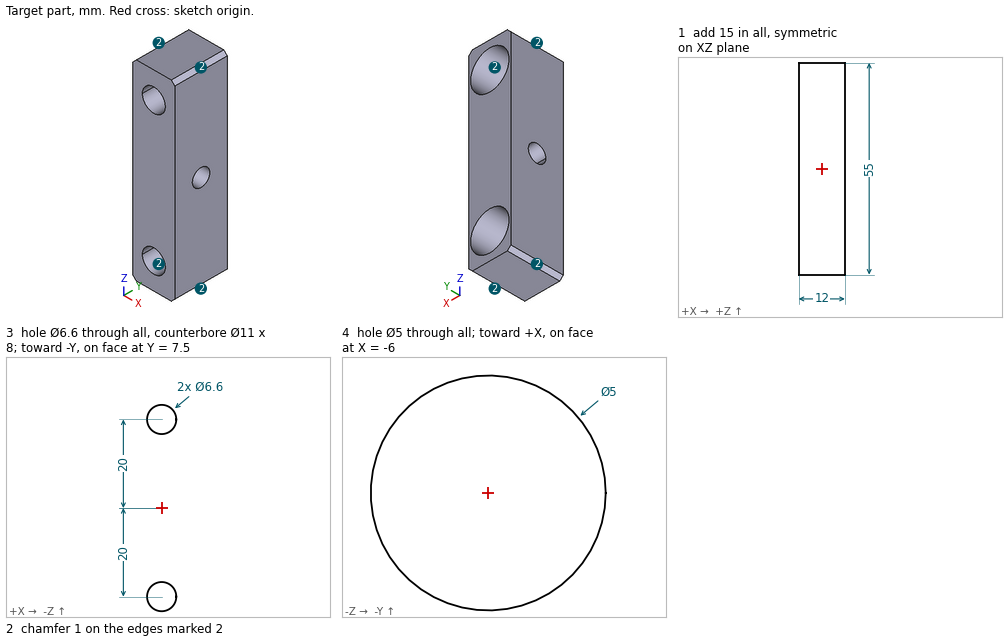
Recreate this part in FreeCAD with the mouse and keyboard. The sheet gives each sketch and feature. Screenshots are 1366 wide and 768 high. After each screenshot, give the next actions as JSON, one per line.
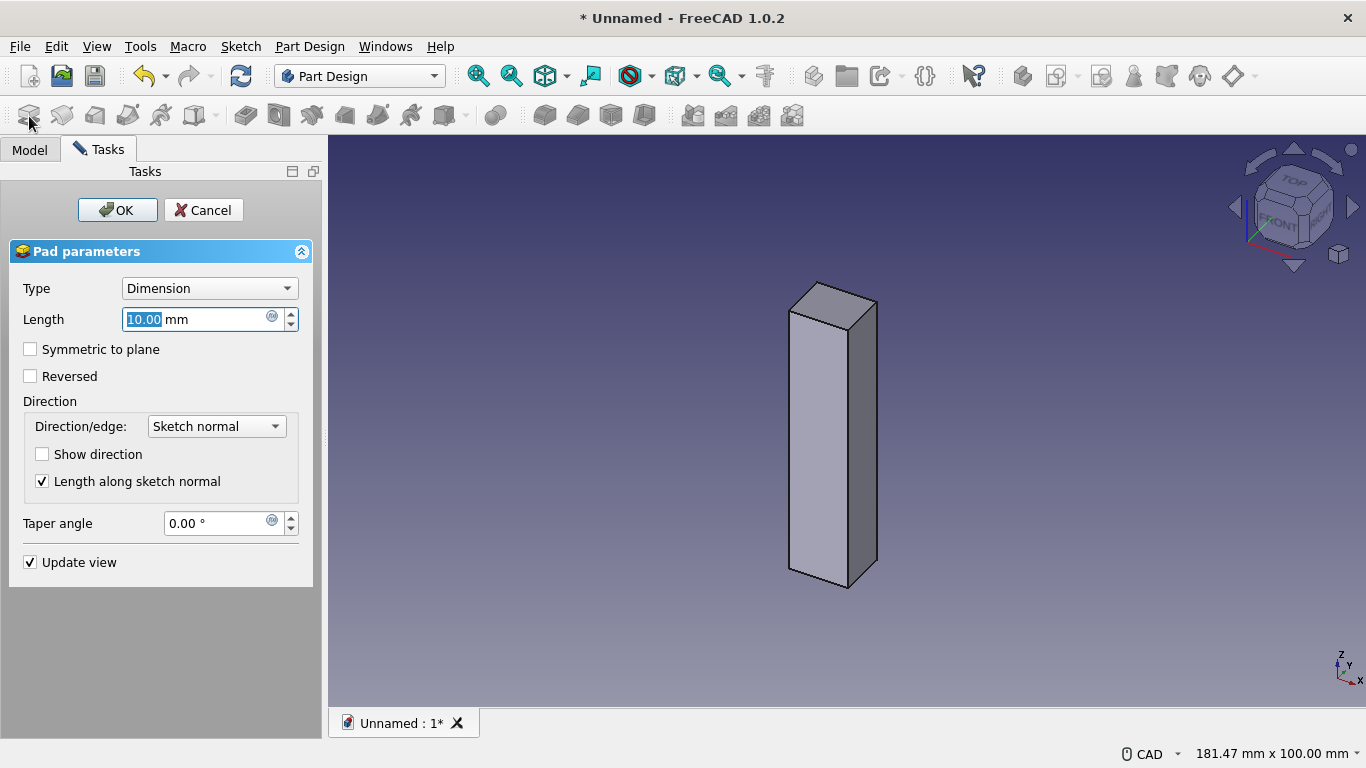
{"action": "type", "text": "15"}
{"action": "key", "text": "Tab"}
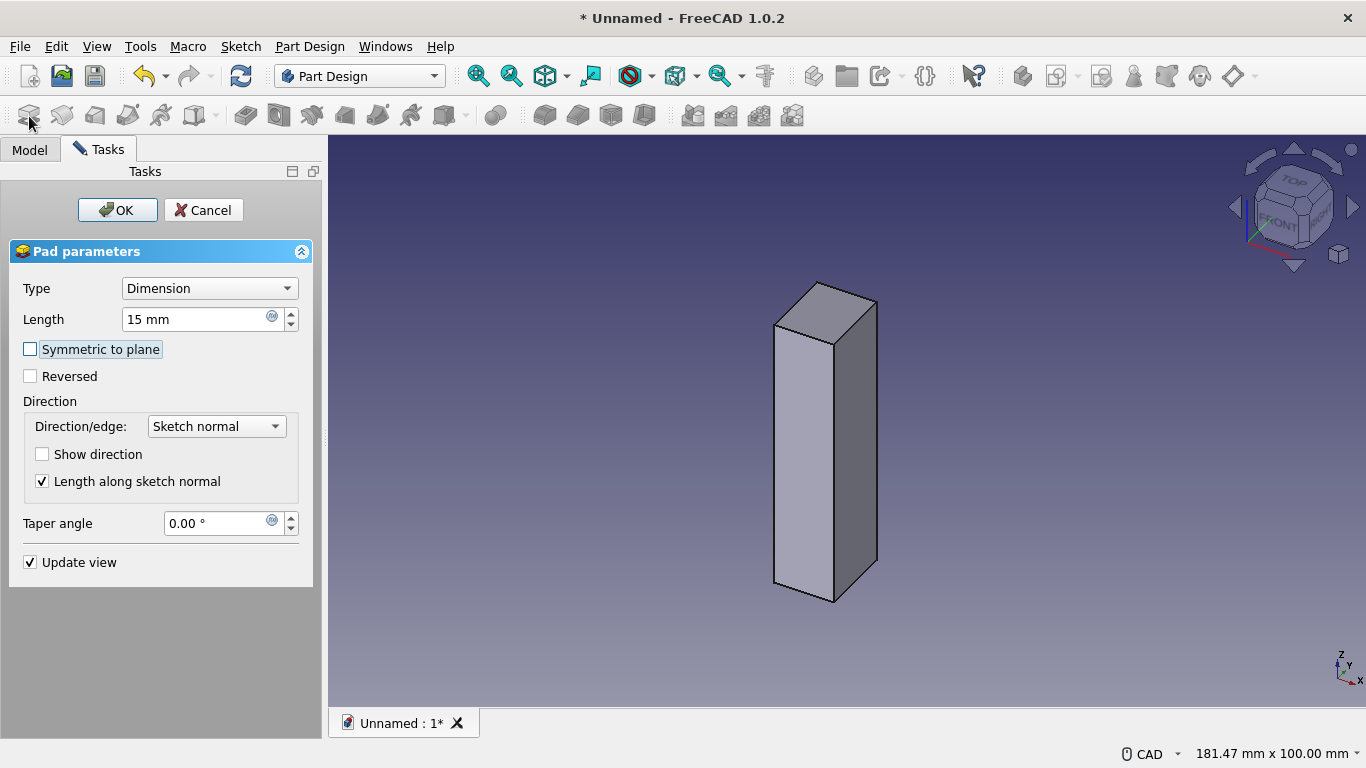
{"action": "left_click", "coordinate": [31, 349]}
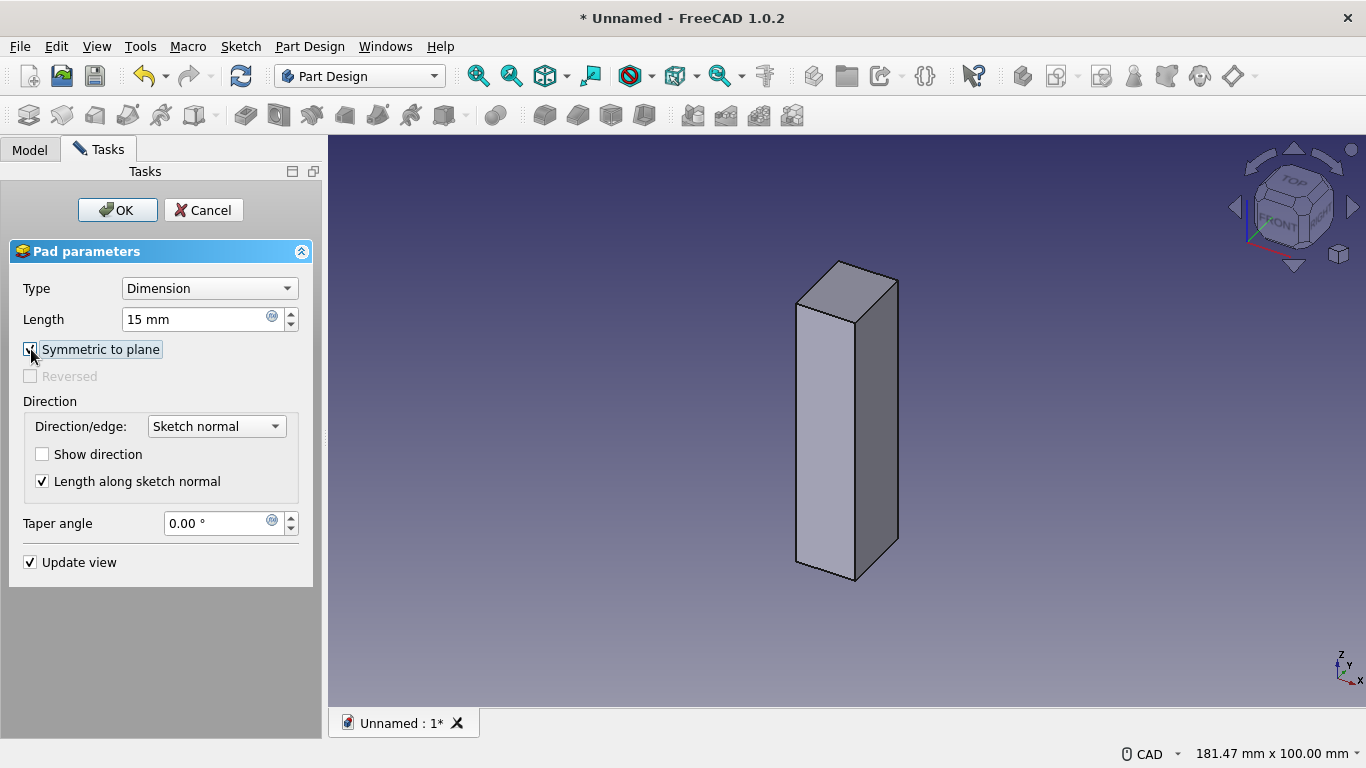
{"action": "left_click", "coordinate": [118, 210]}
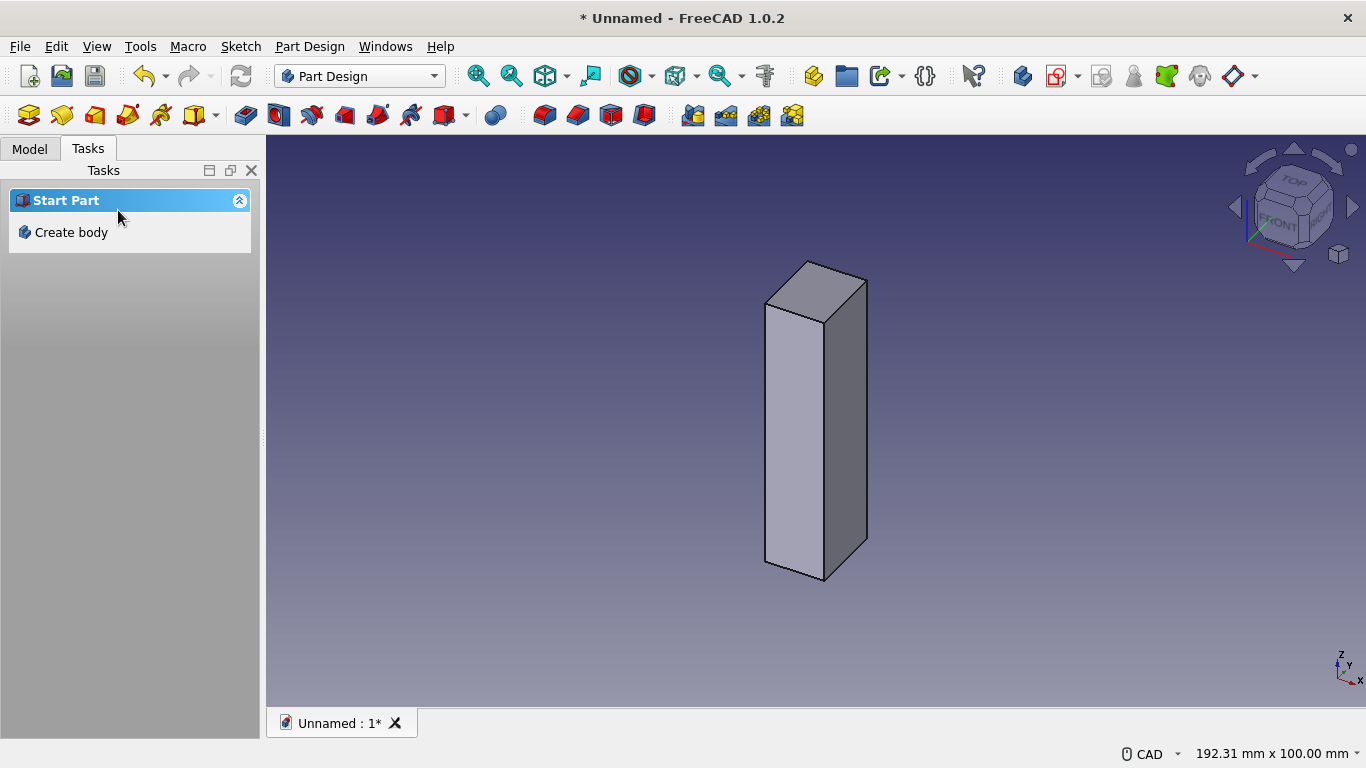
{"action": "left_click", "coordinate": [846, 301]}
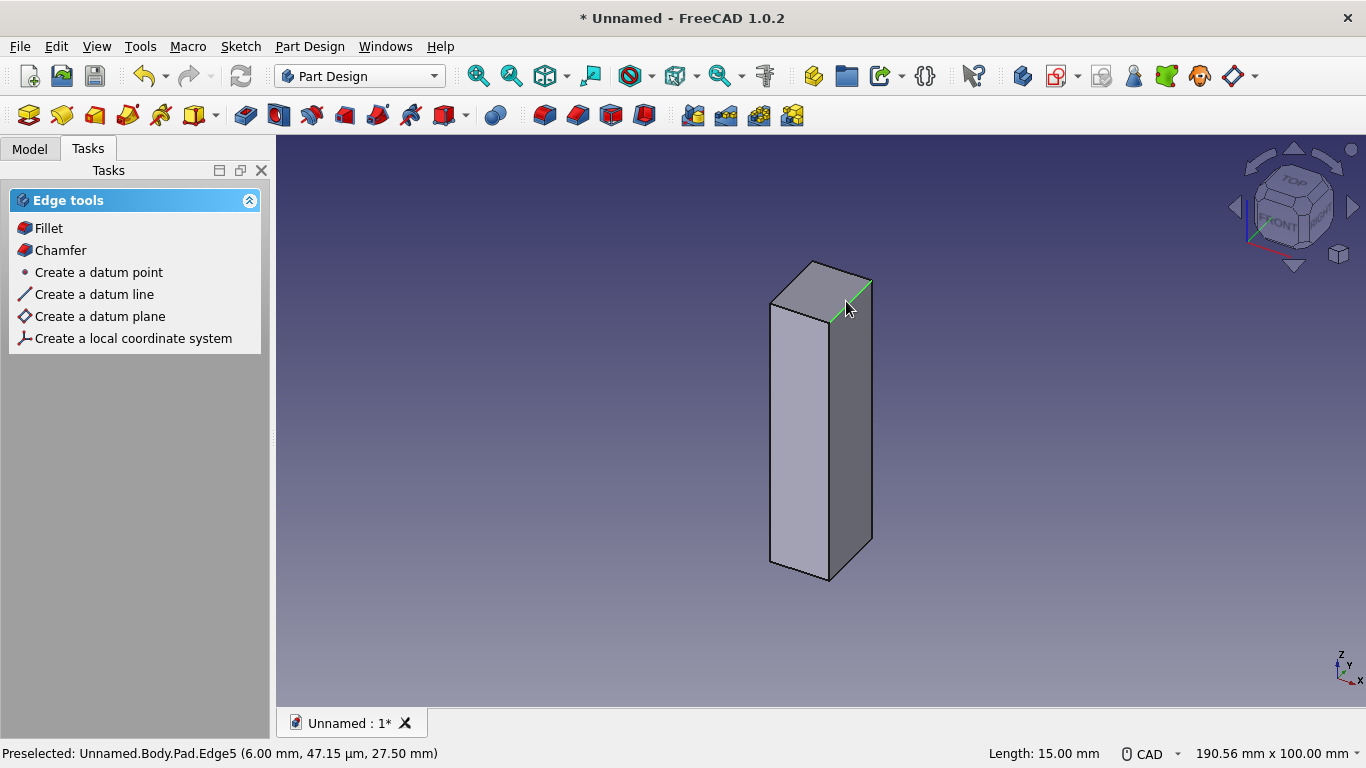
{"action": "key", "text": "0"}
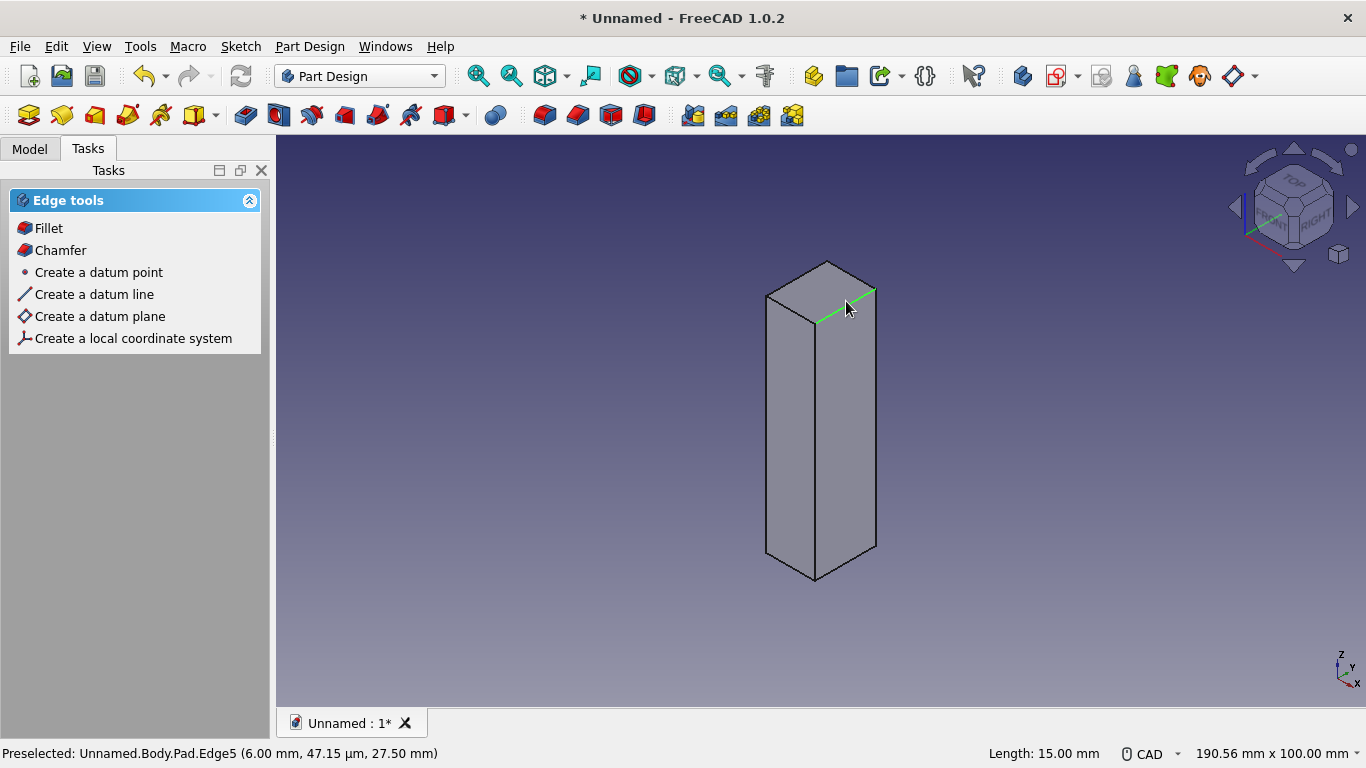
{"action": "key", "text": "2"}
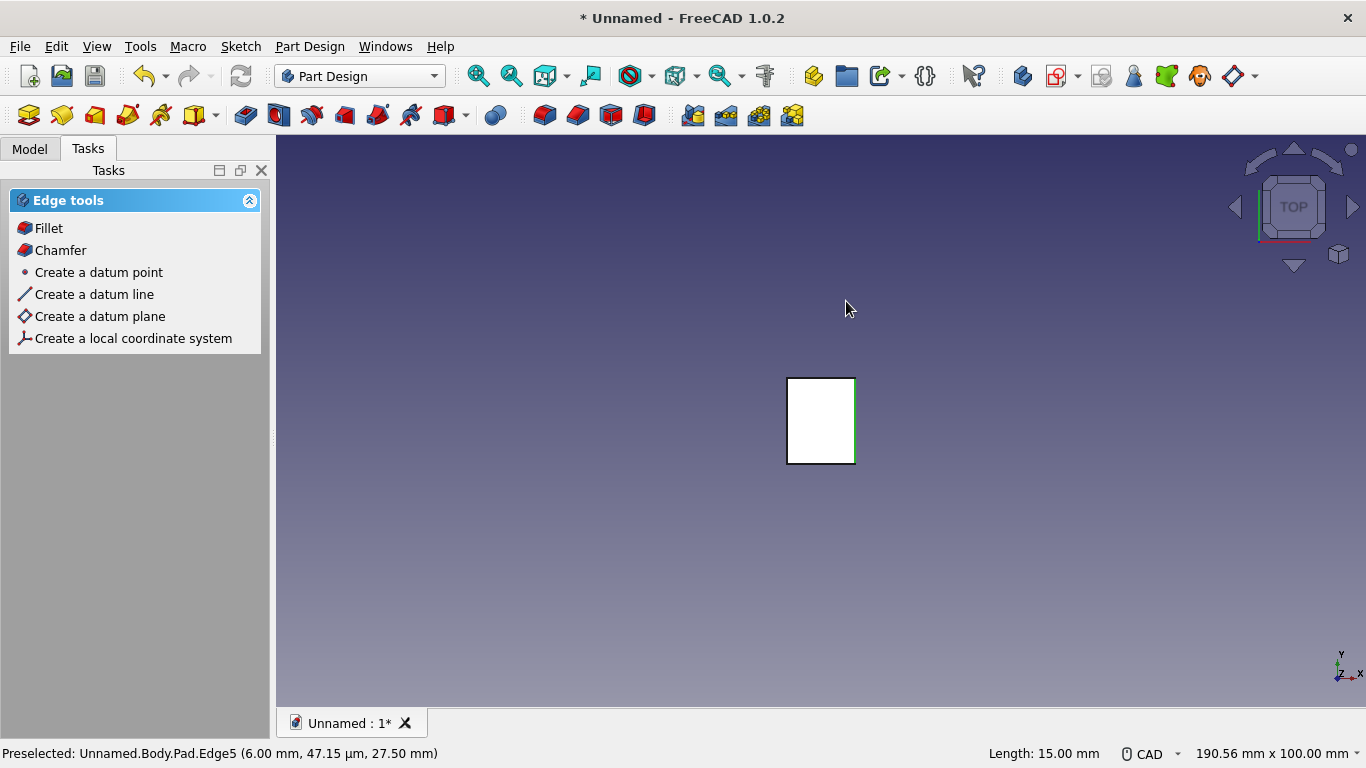
{"action": "left_click", "coordinate": [479, 76]}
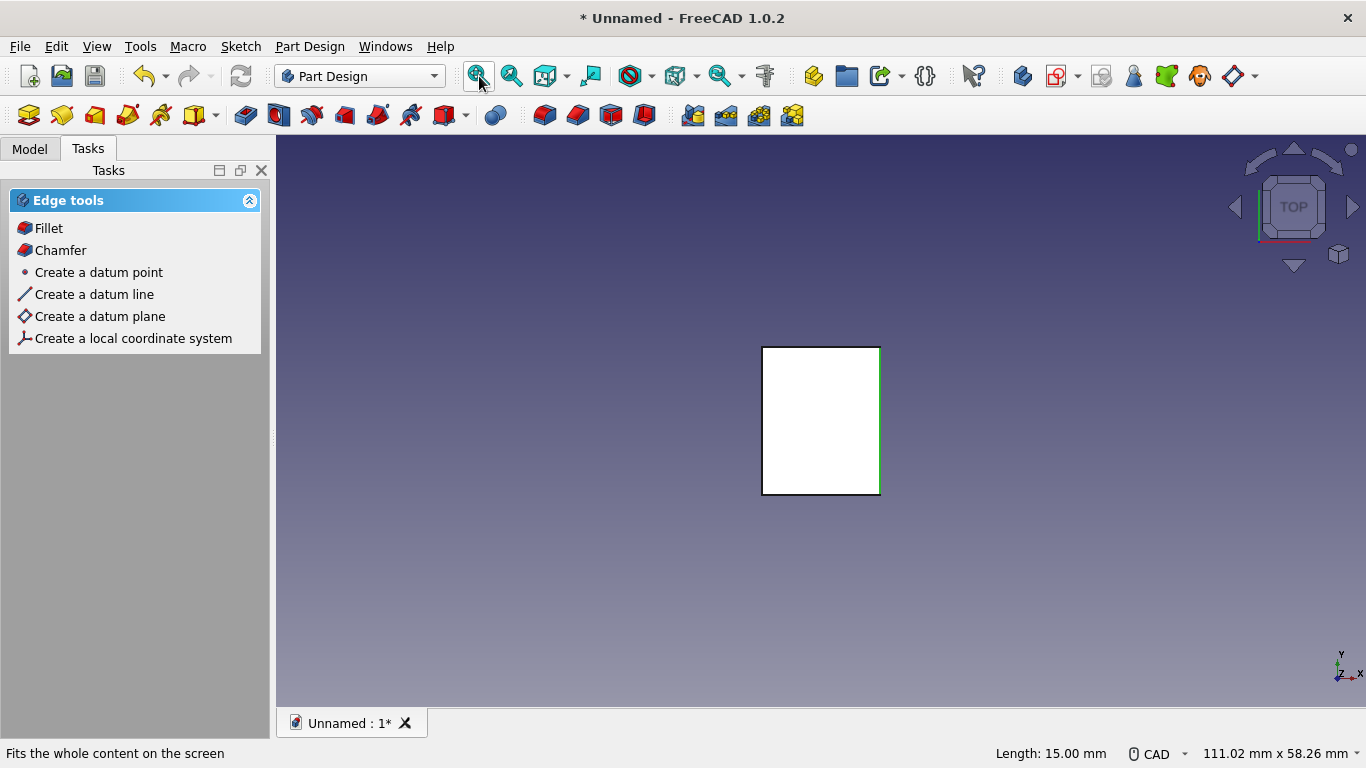
{"action": "left_click", "coordinate": [762, 420], "text": "ctrl"}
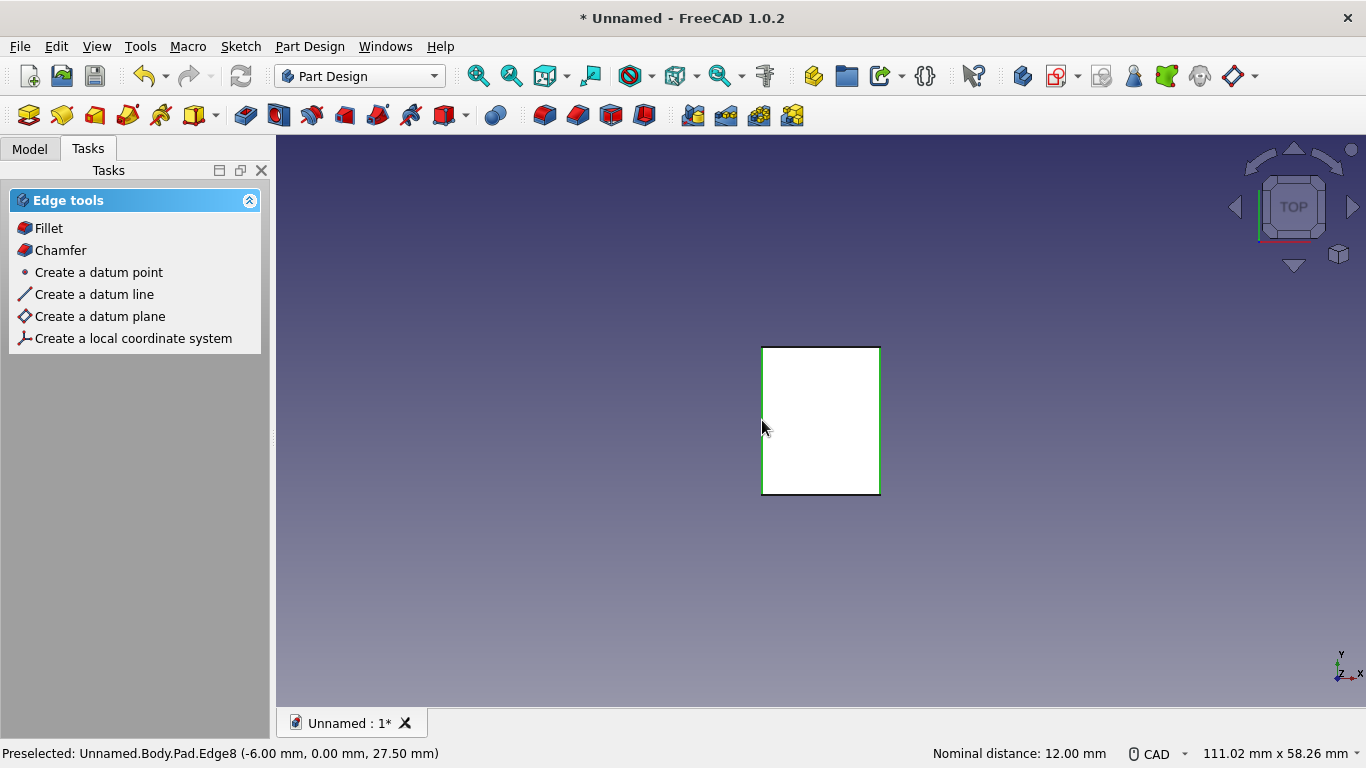
{"action": "key", "text": "1"}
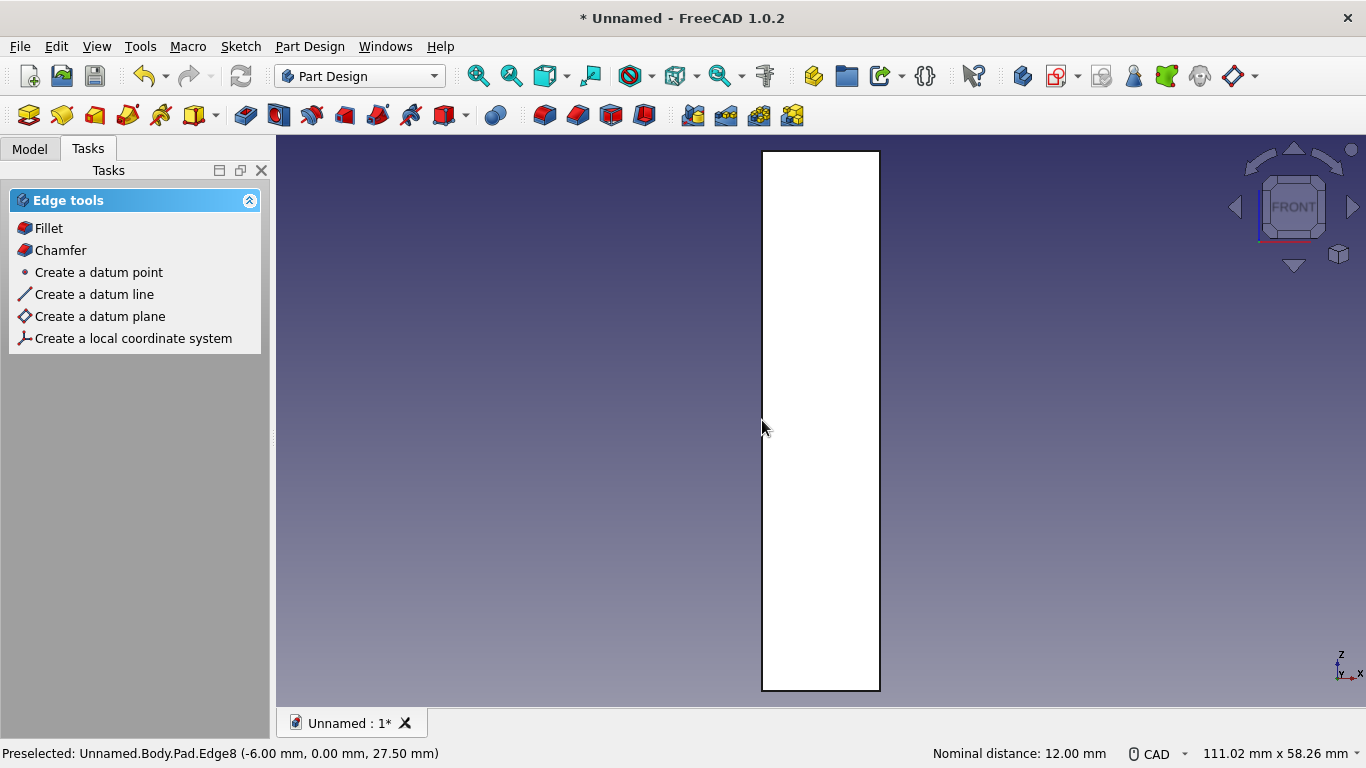
{"action": "key", "text": "3"}